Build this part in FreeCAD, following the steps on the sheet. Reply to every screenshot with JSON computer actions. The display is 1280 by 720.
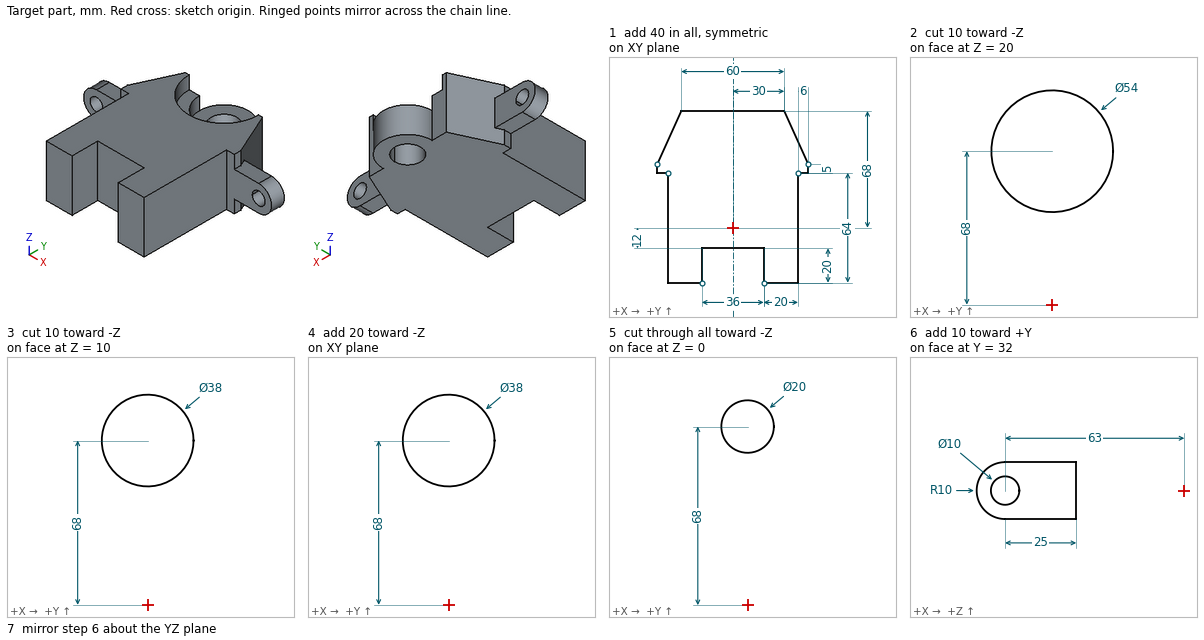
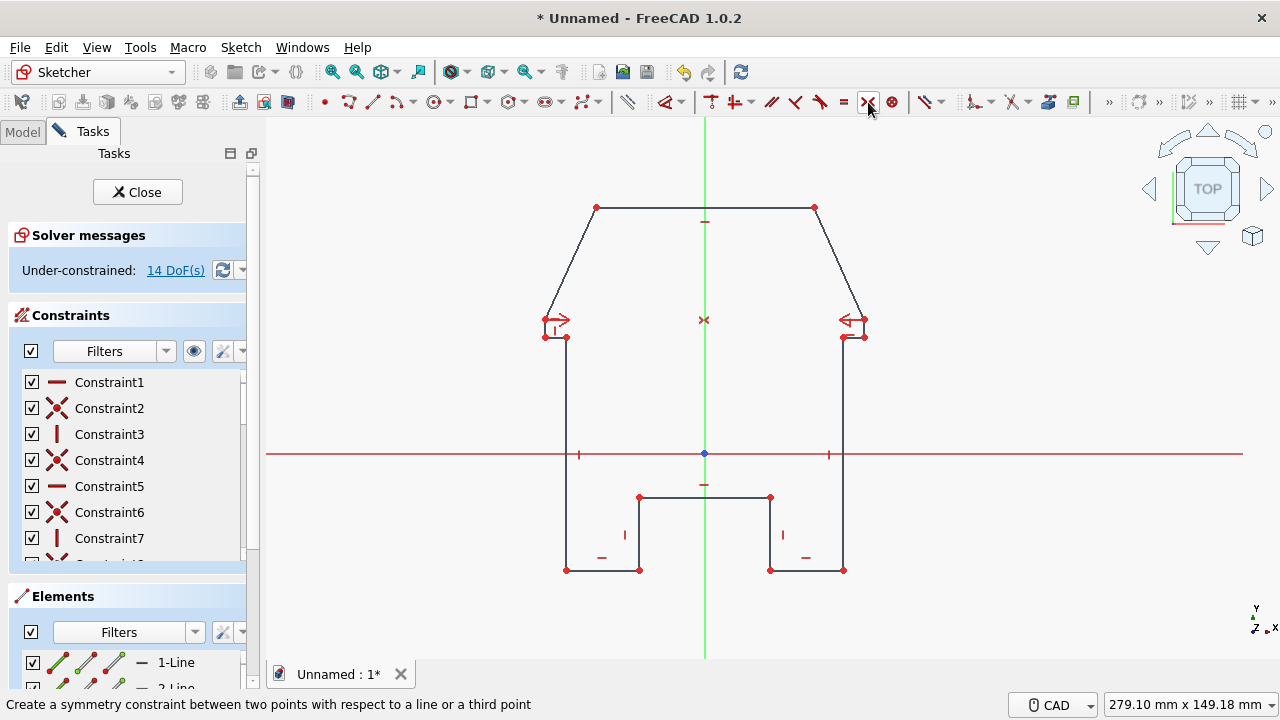
{"action": "left_click", "coordinate": [843, 338]}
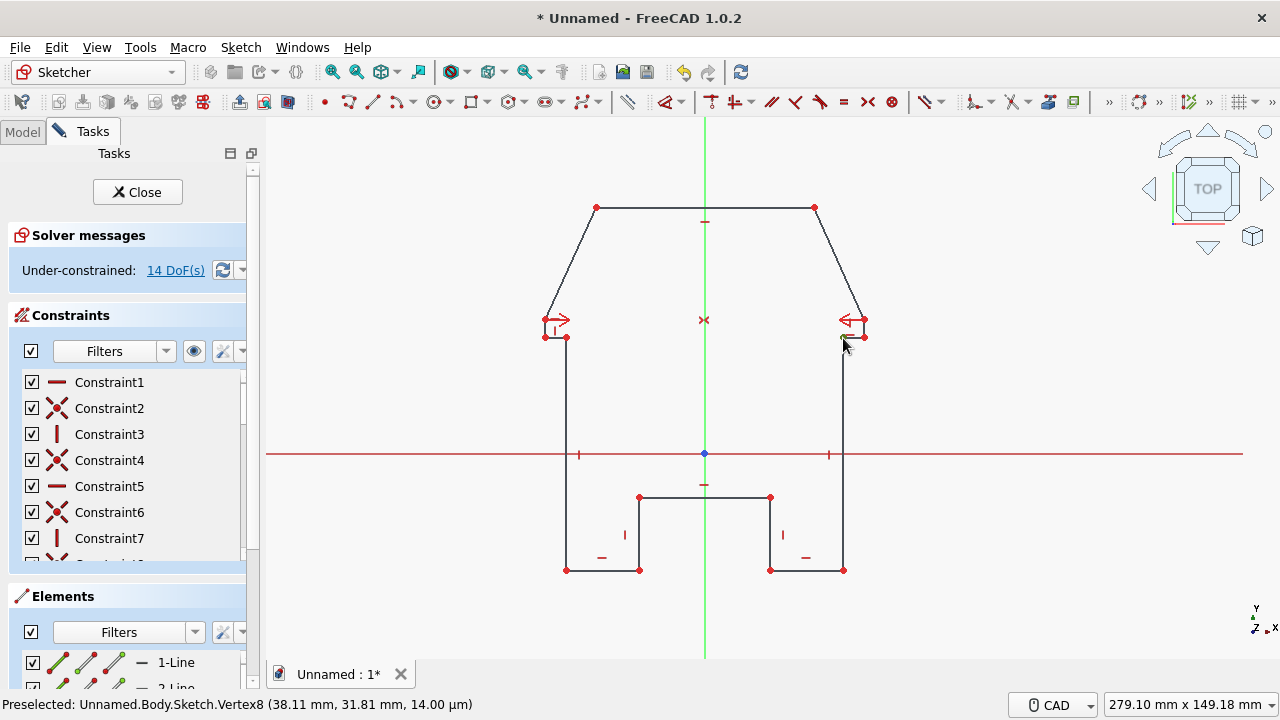
{"action": "left_click", "coordinate": [566, 338]}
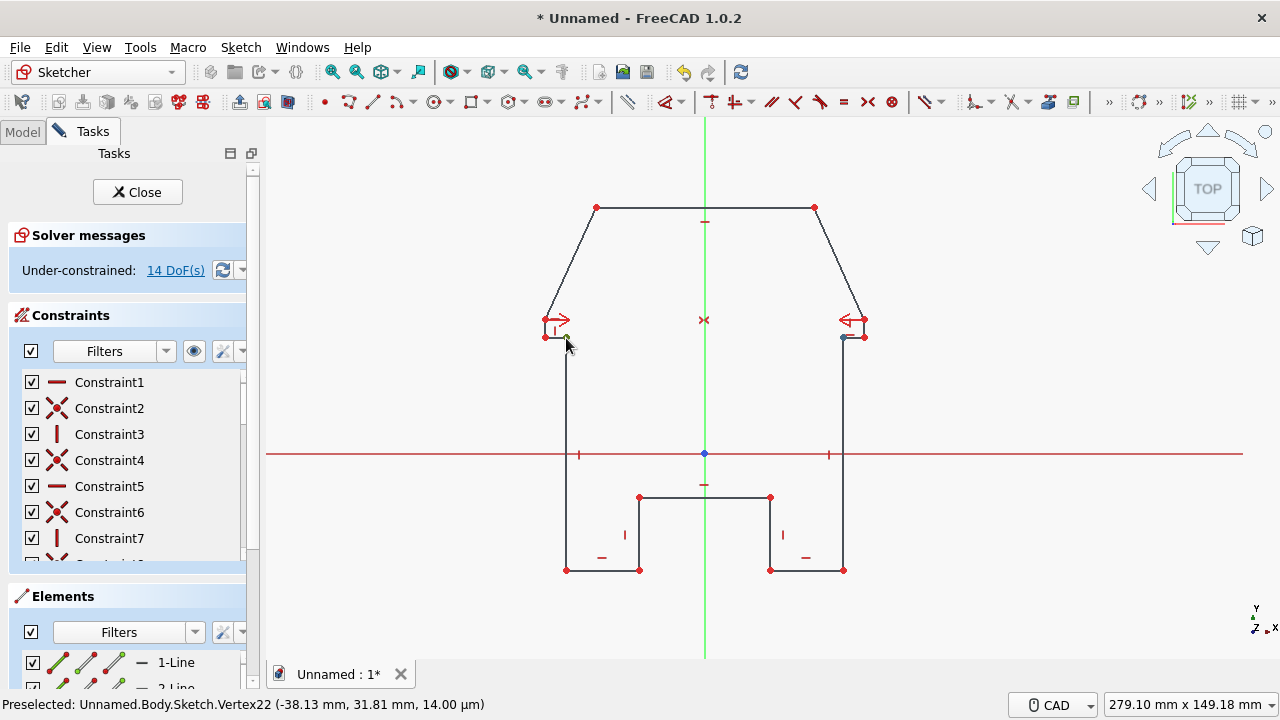
{"action": "left_click", "coordinate": [705, 596]}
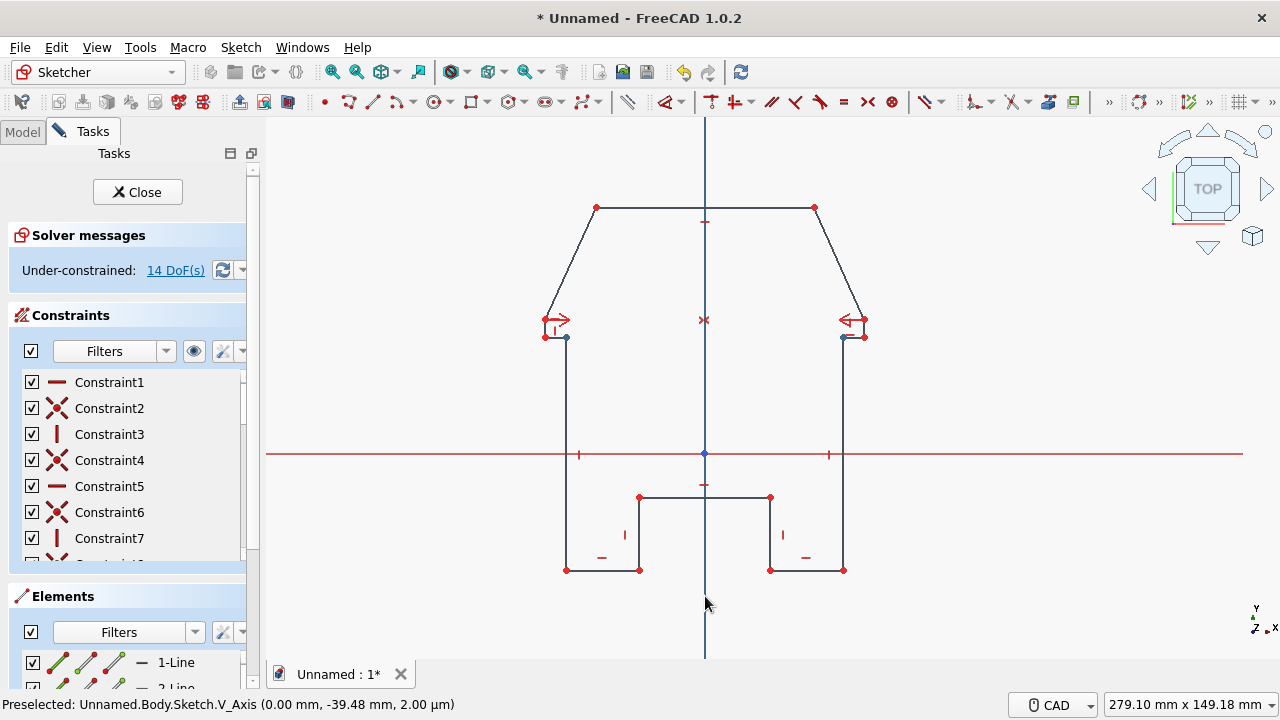
{"action": "left_click", "coordinate": [868, 102]}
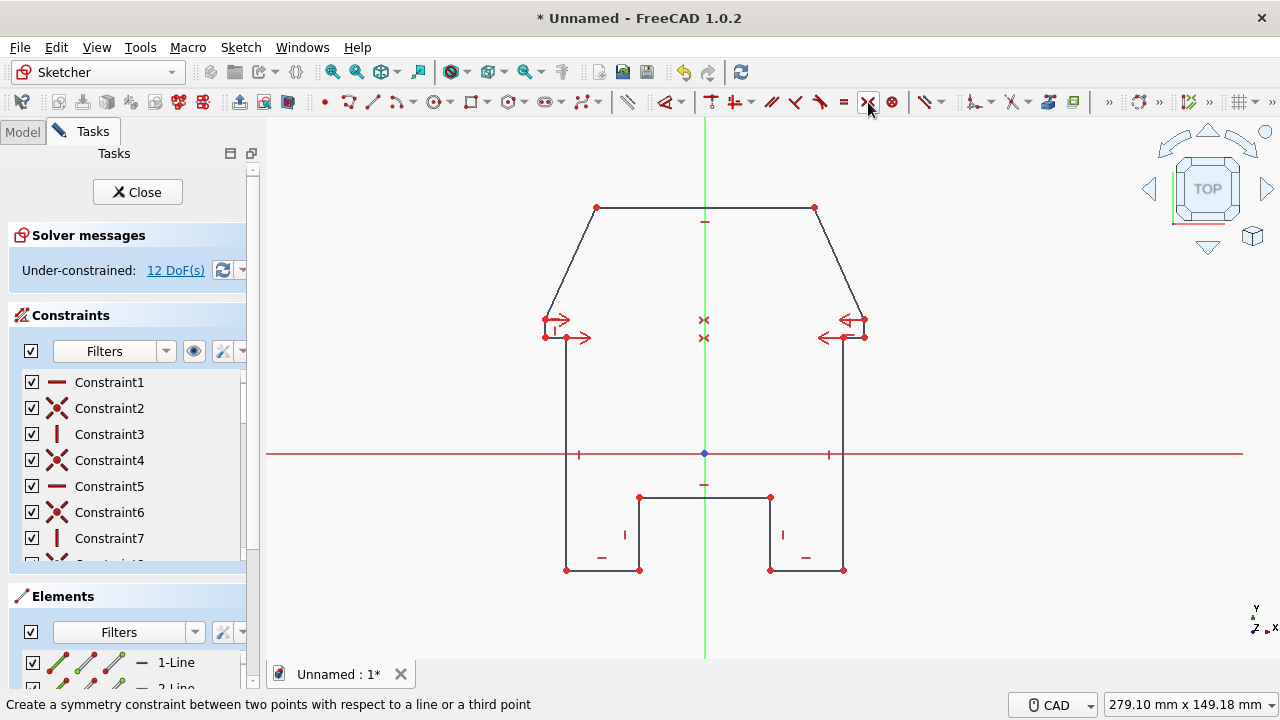
{"action": "left_click", "coordinate": [770, 571]}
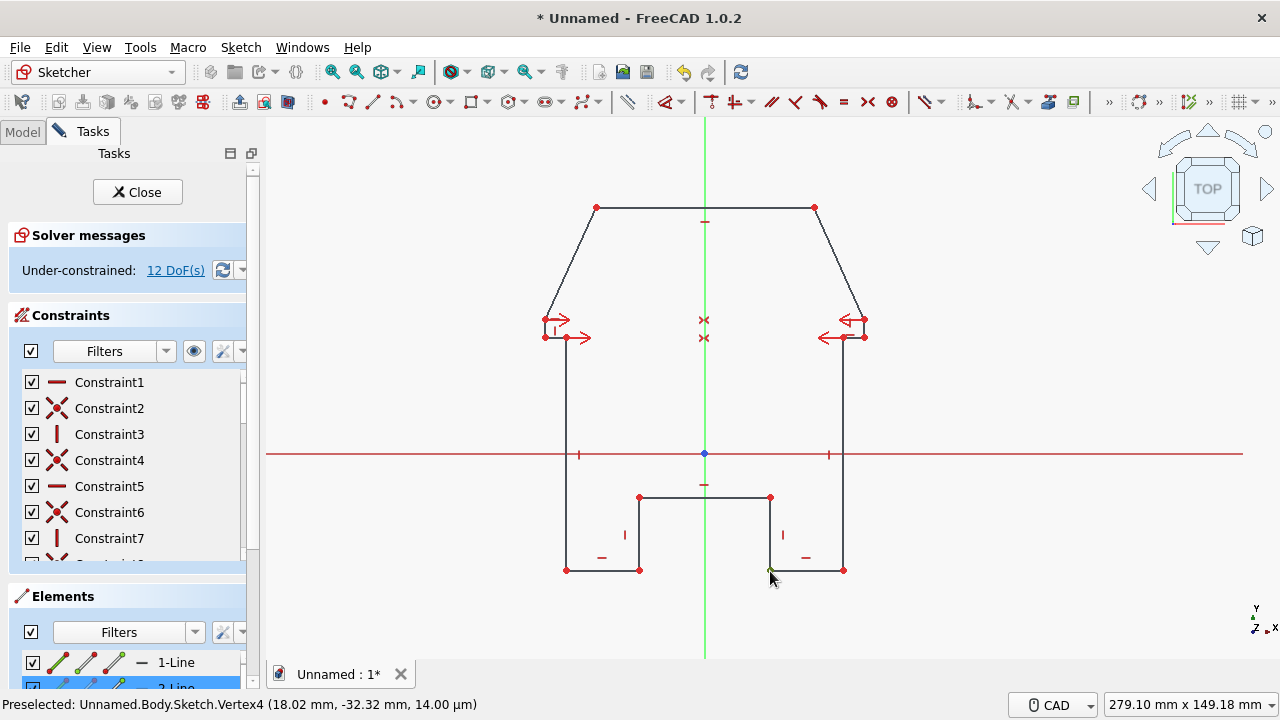
{"action": "left_click", "coordinate": [639, 571]}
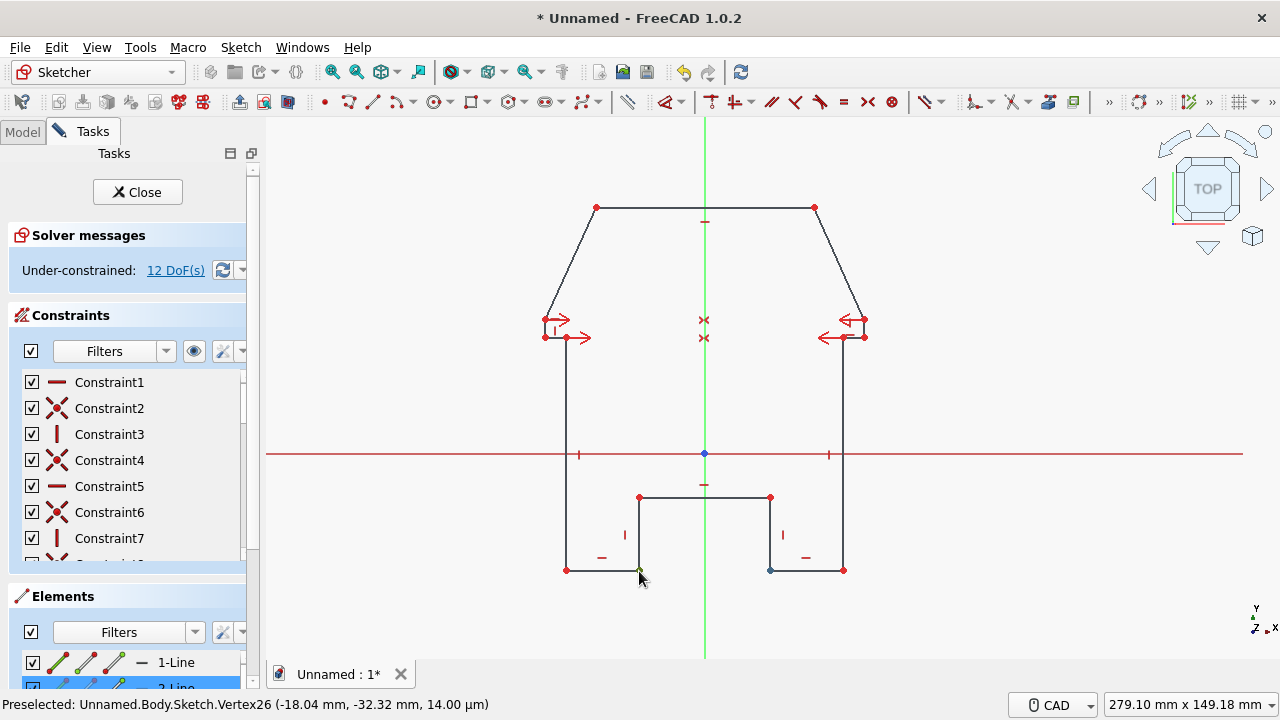
{"action": "left_click", "coordinate": [705, 596]}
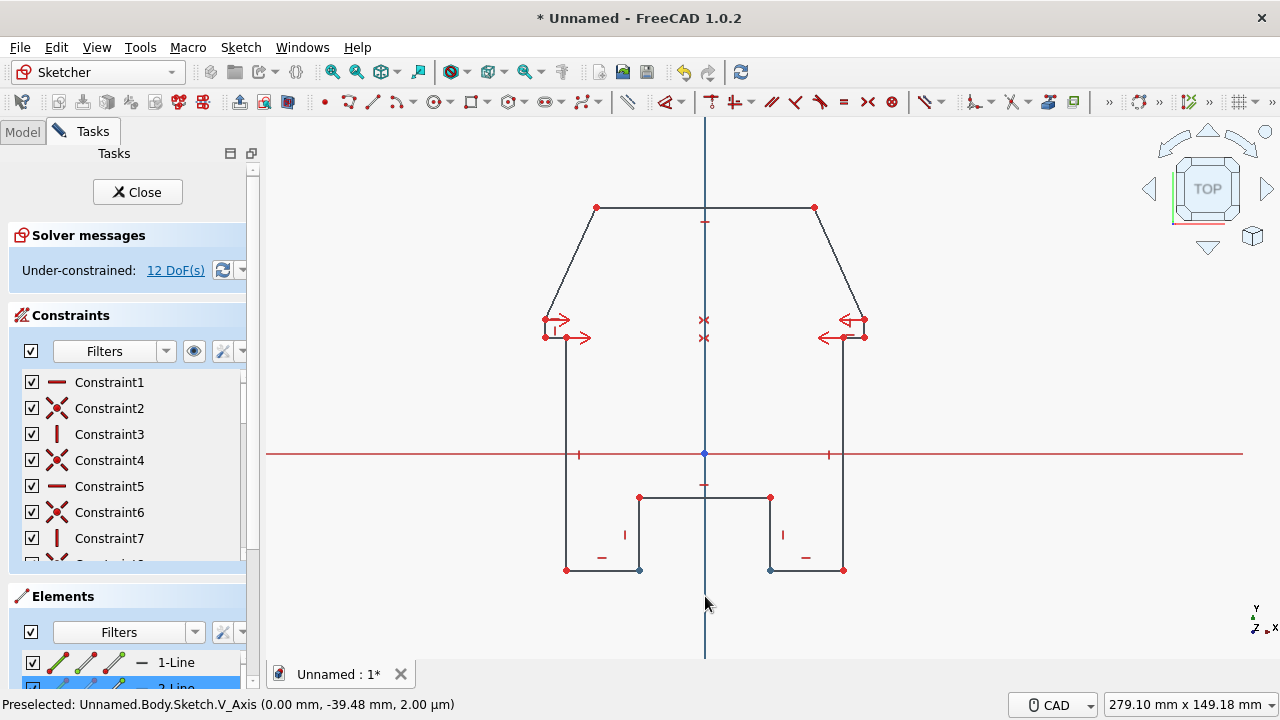
{"action": "left_click", "coordinate": [868, 102]}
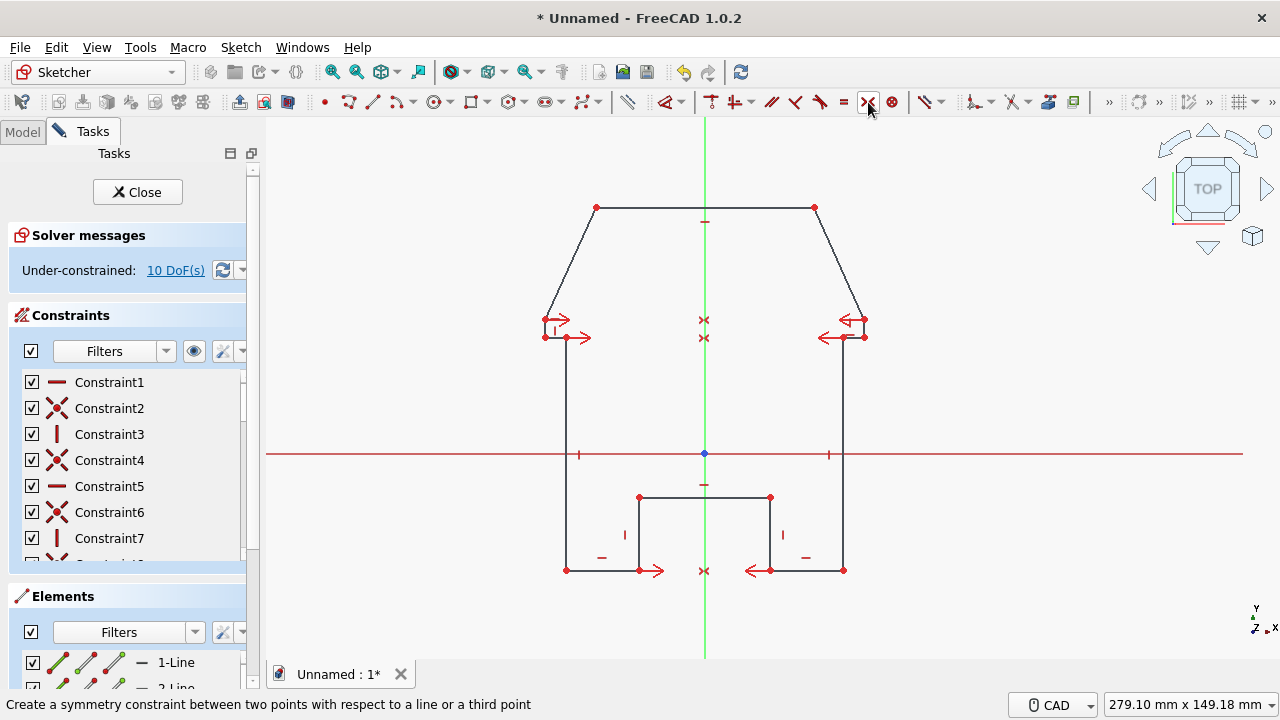
{"action": "scroll", "coordinate": [854, 338], "scroll_direction": "up", "scroll_amount": 3}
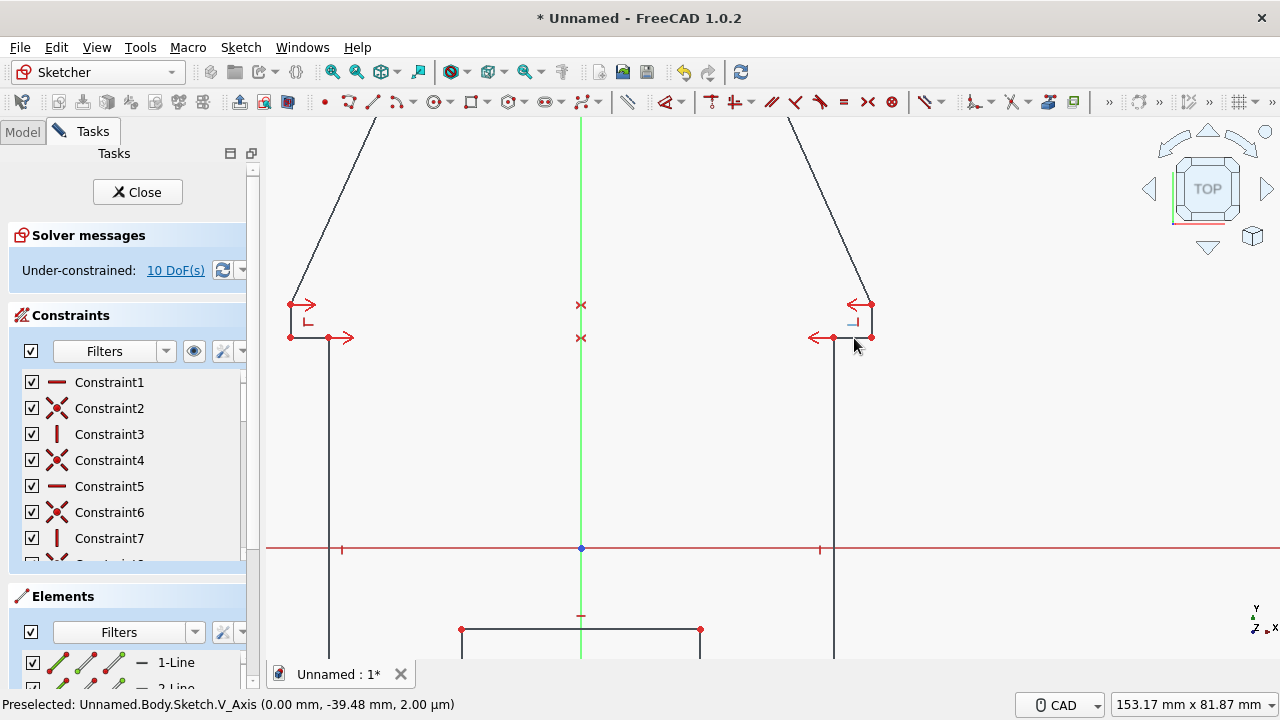
{"action": "left_click", "coordinate": [853, 338]}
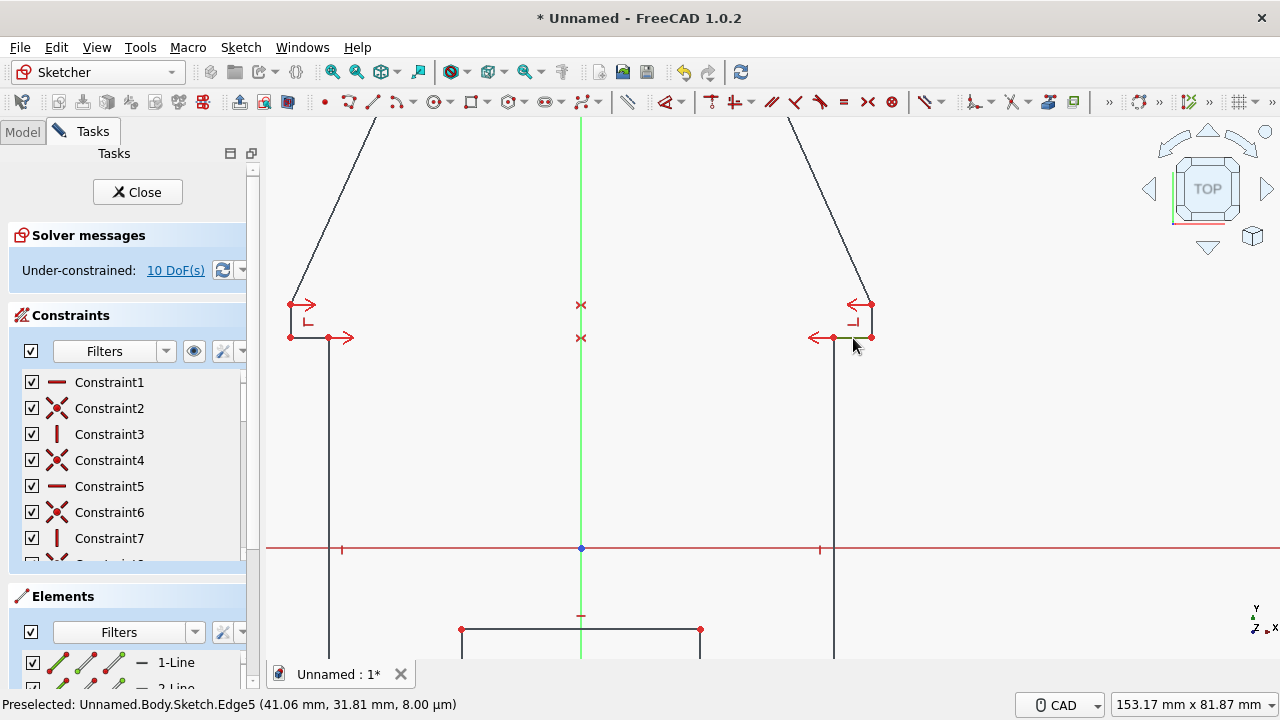
{"action": "key", "text": "l"}